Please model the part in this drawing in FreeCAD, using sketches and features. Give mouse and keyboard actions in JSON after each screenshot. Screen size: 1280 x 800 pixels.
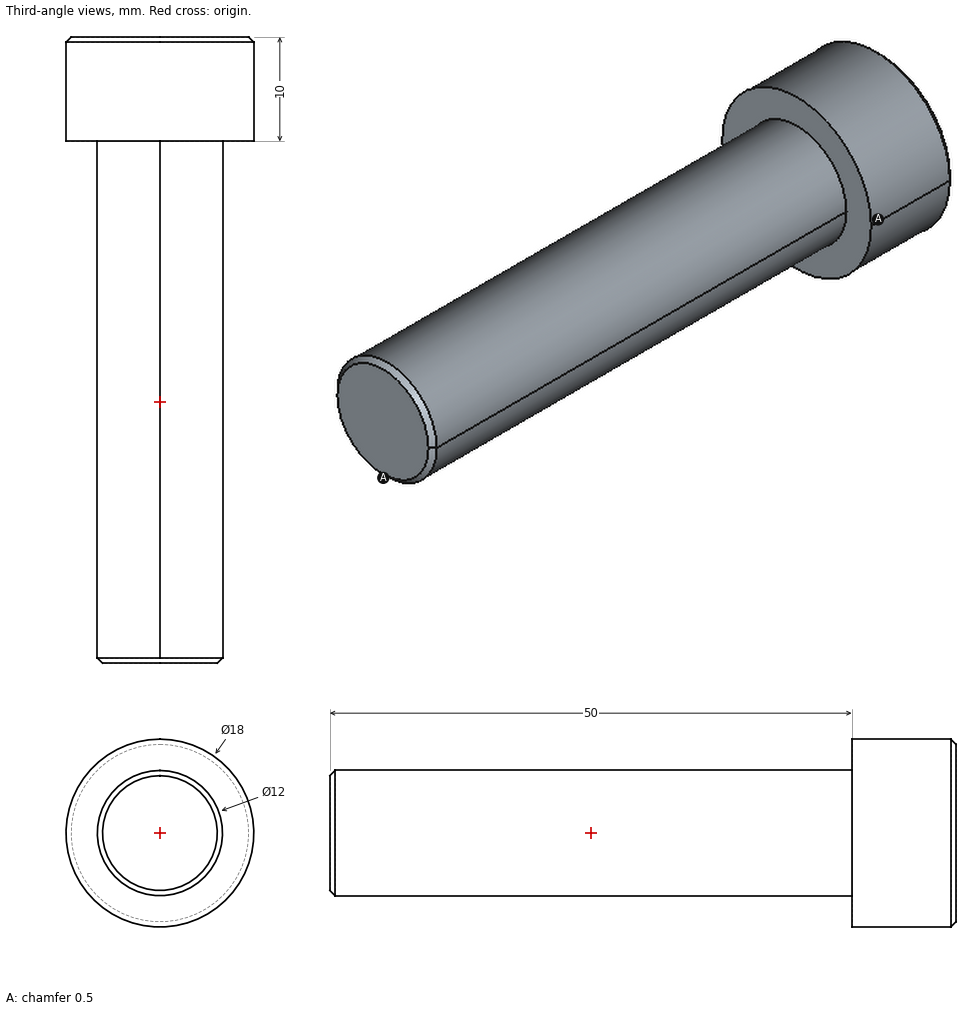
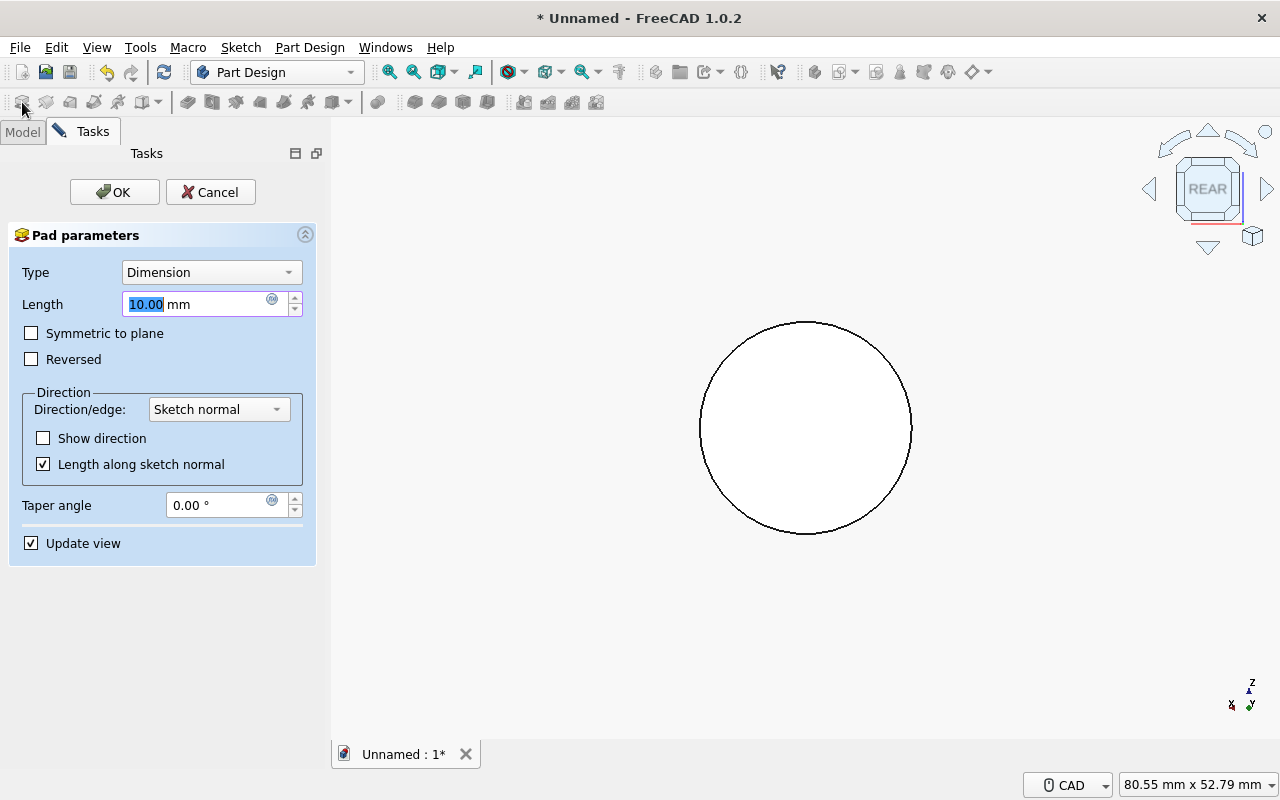
{"action": "type", "text": "10"}
{"action": "key", "text": "Tab"}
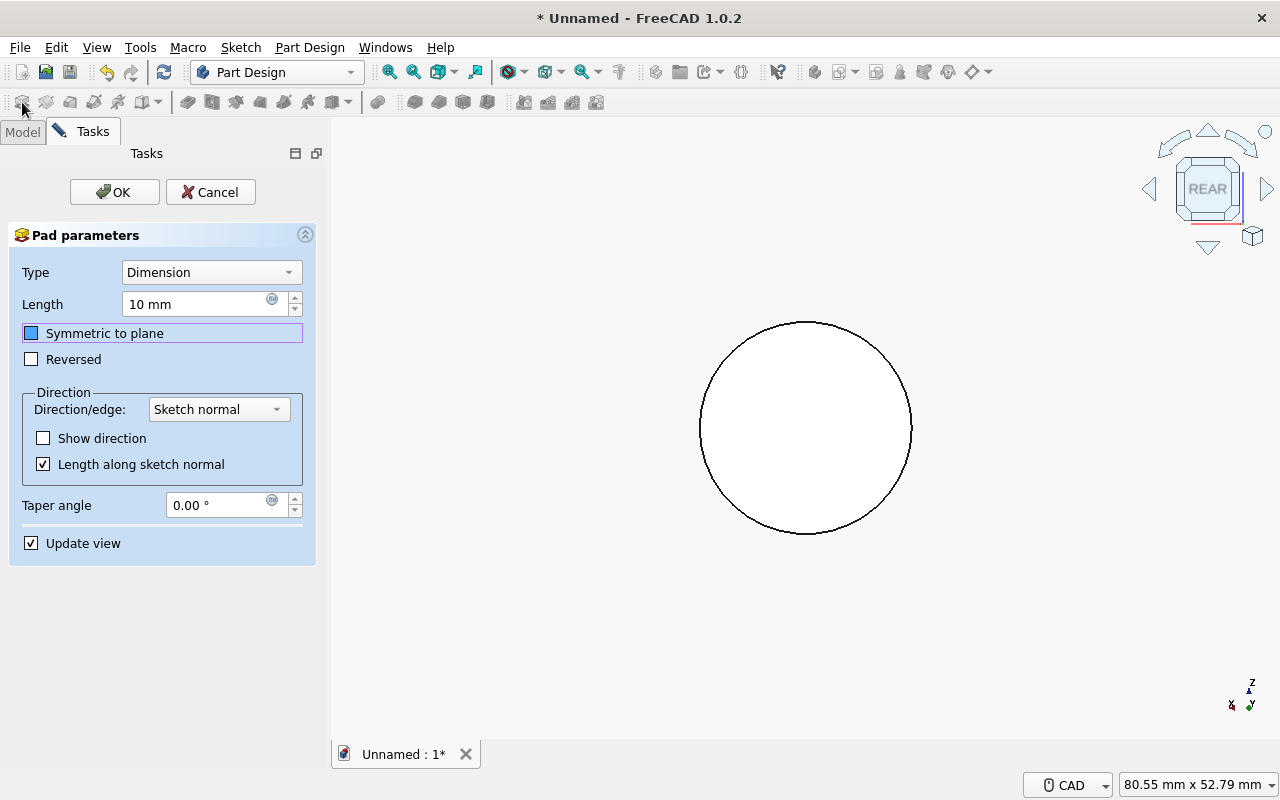
{"action": "left_click", "coordinate": [115, 192]}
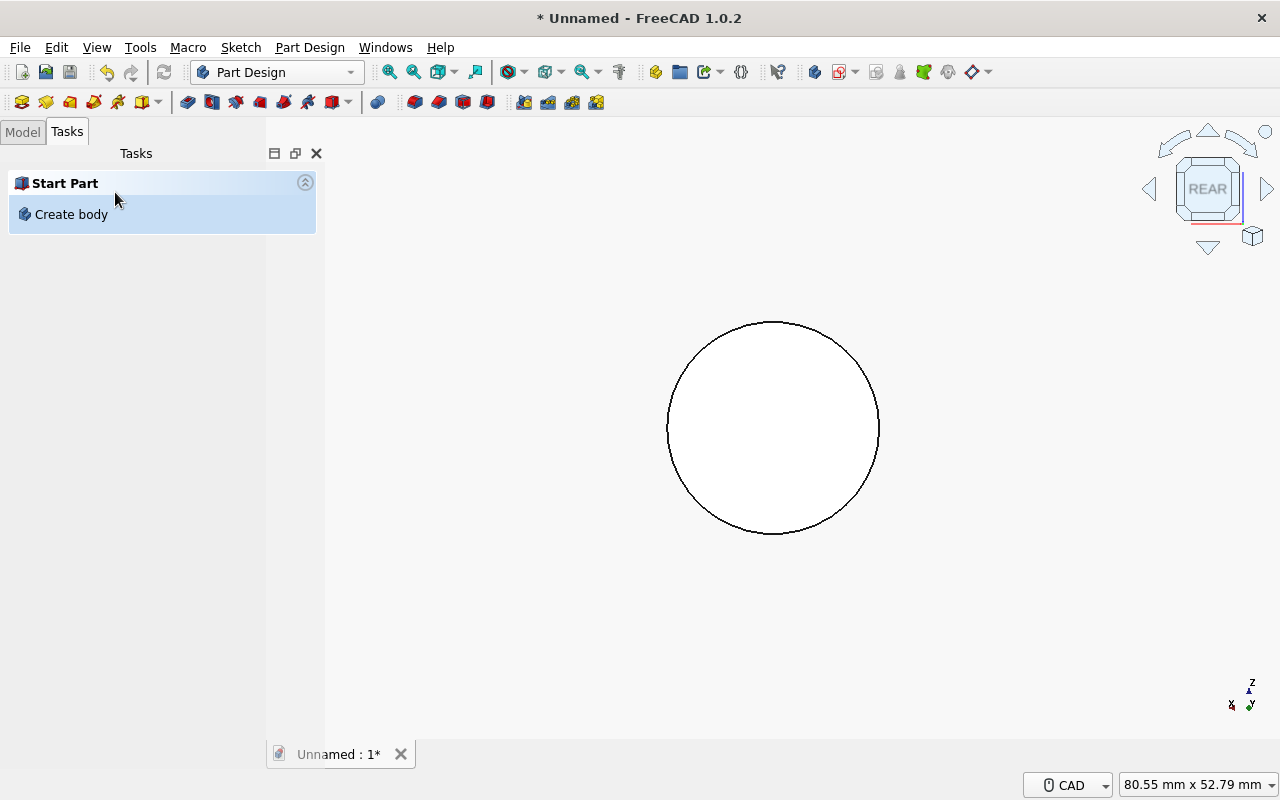
{"action": "left_click", "coordinate": [390, 72]}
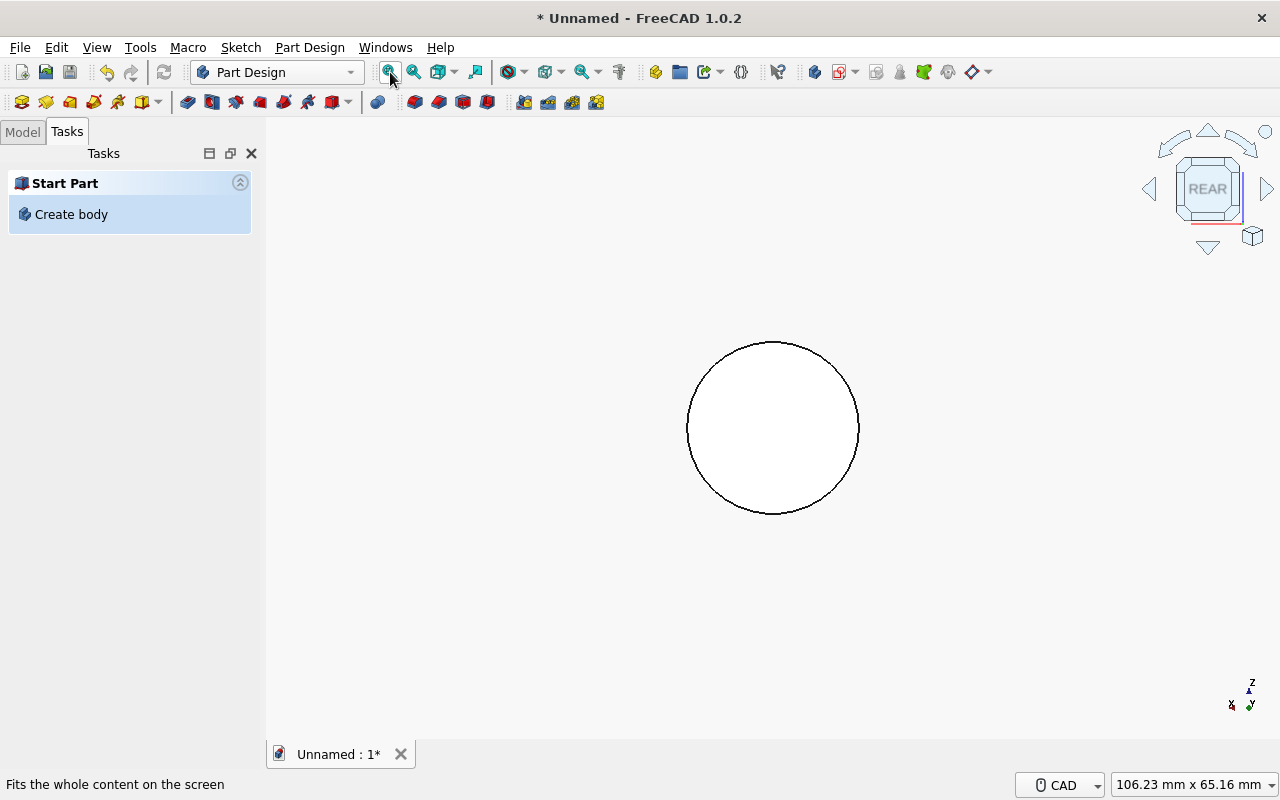
{"action": "left_click", "coordinate": [859, 427]}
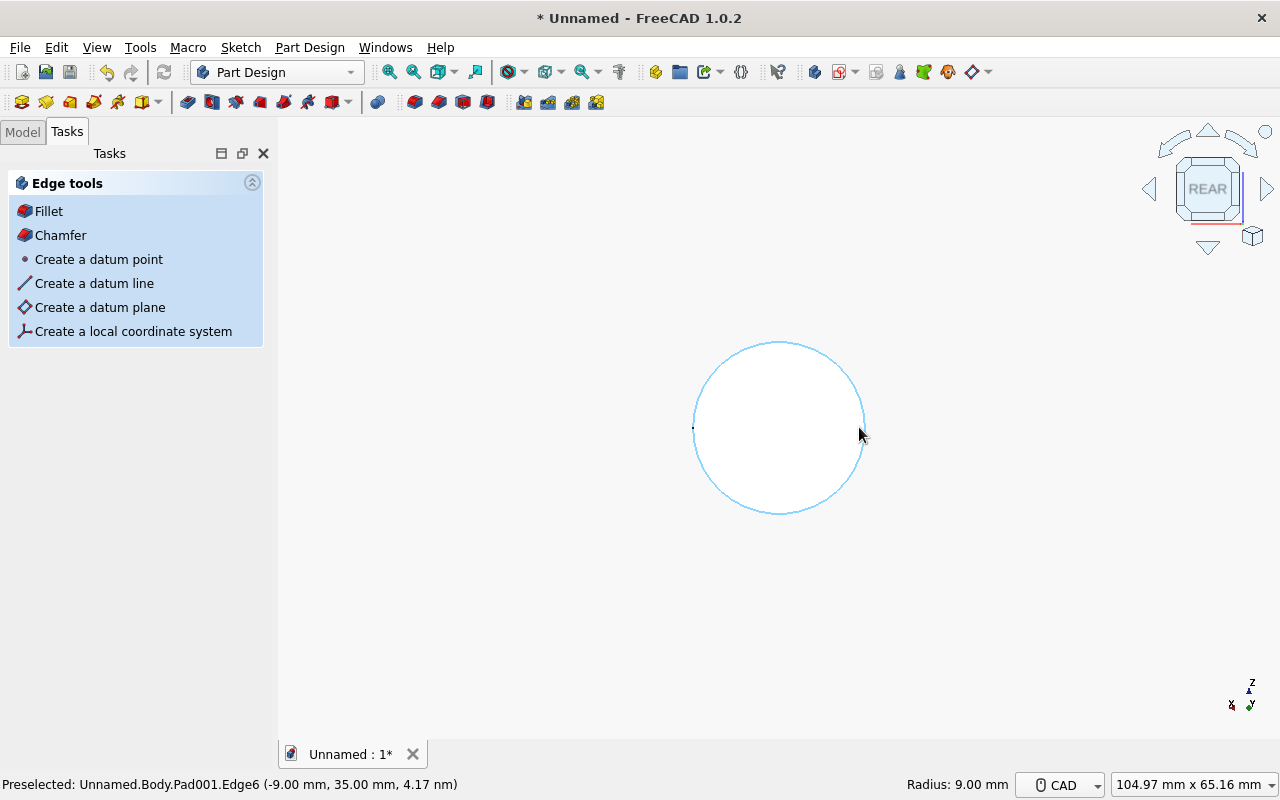
{"action": "key", "text": "0"}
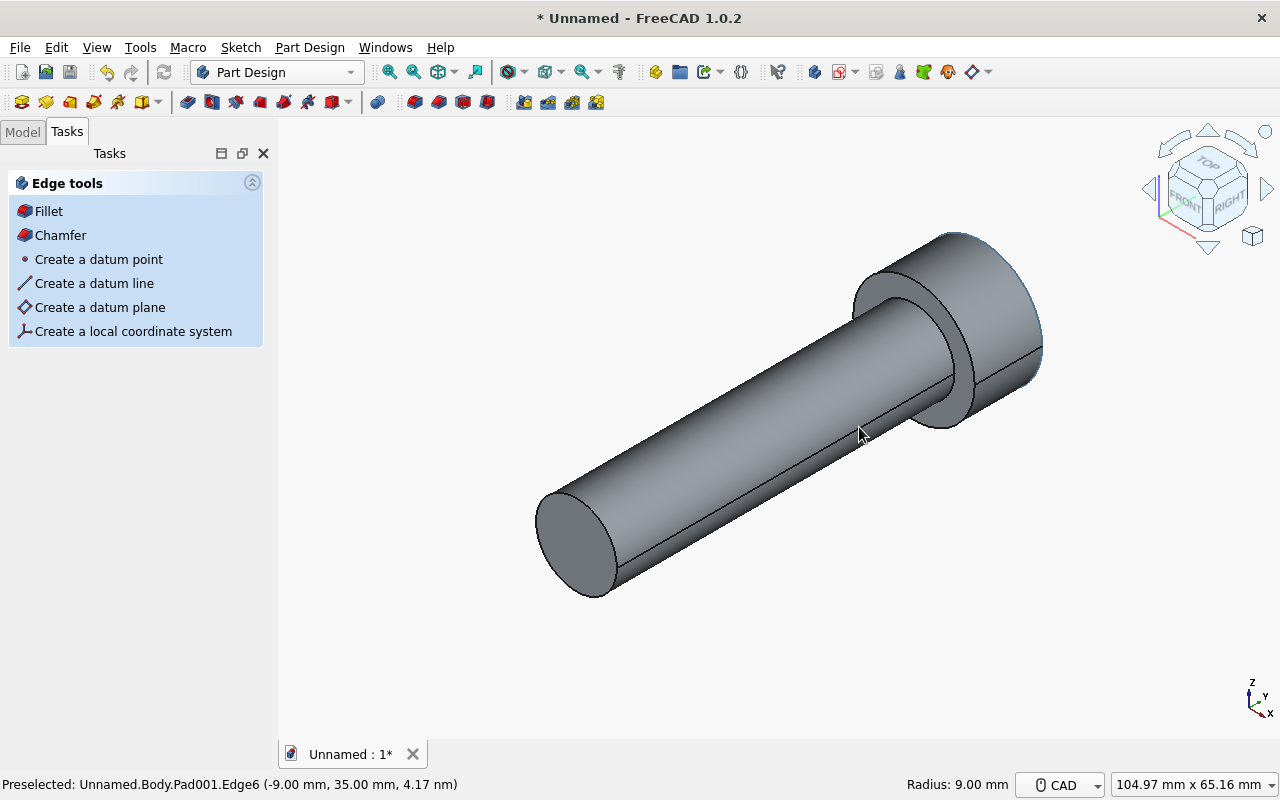
{"action": "left_click", "coordinate": [564, 492], "text": "ctrl"}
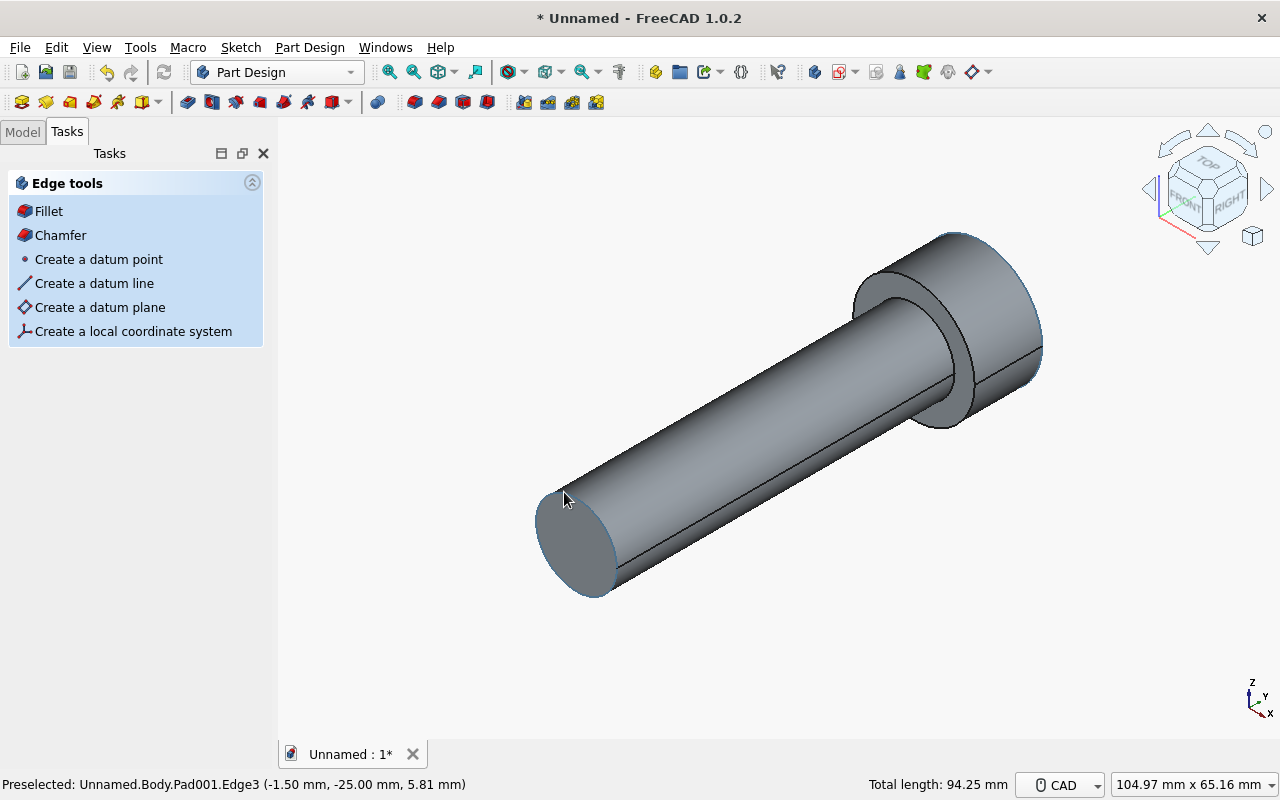
{"action": "left_click", "coordinate": [440, 102]}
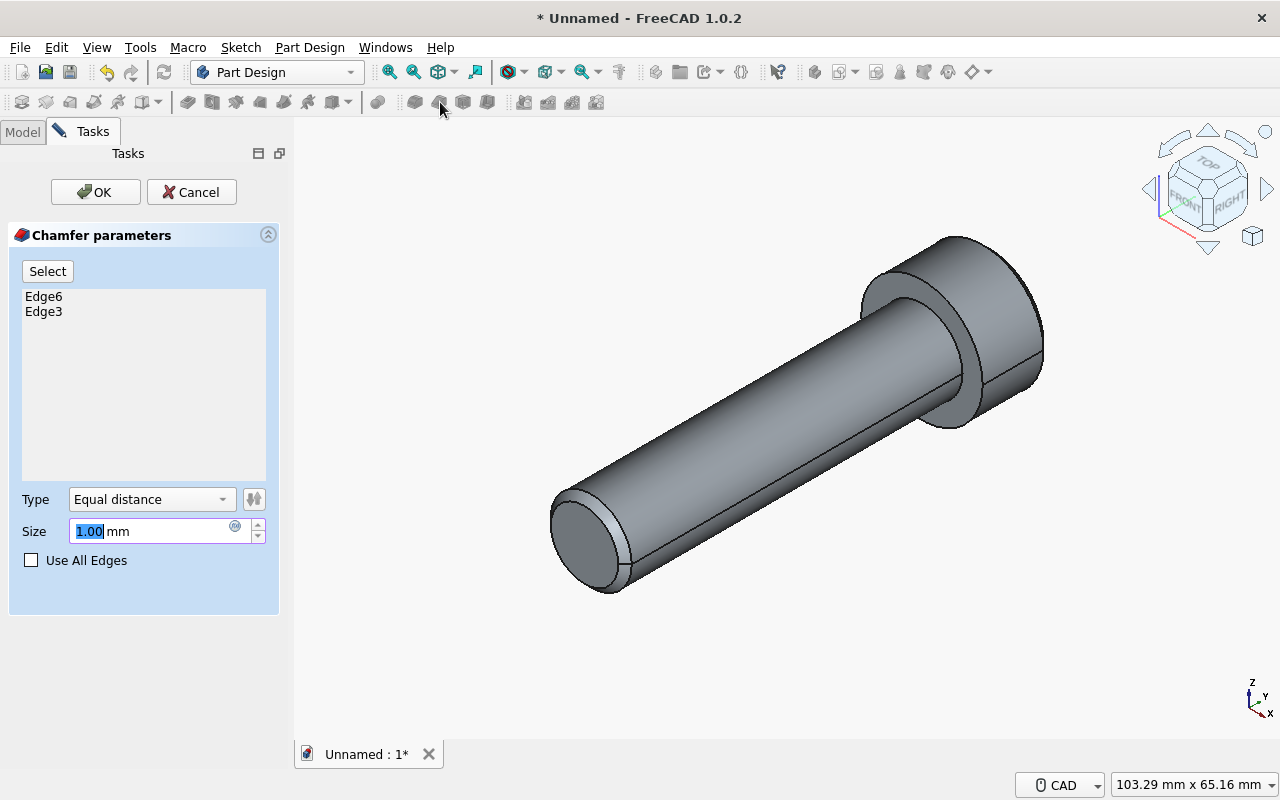
{"action": "type", "text": "0.5"}
{"action": "key", "text": "Tab"}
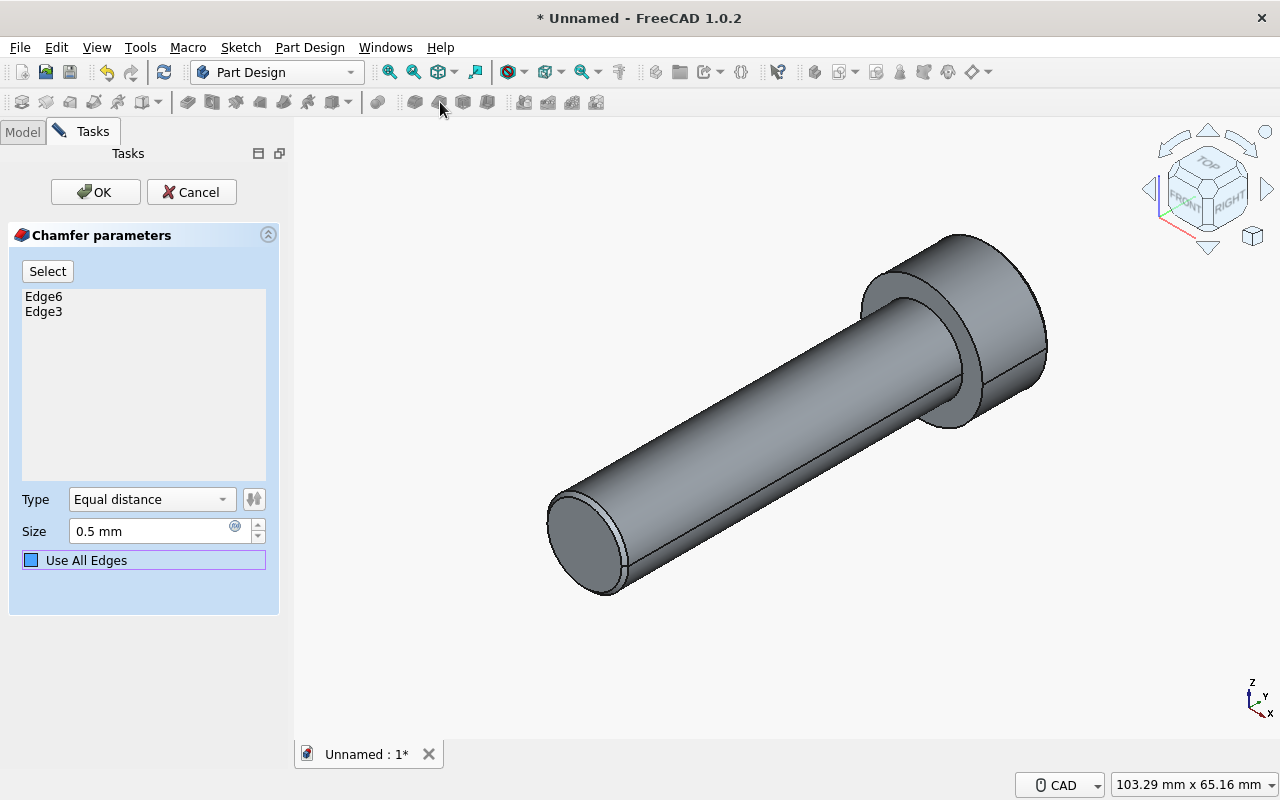
{"action": "left_click", "coordinate": [96, 192]}